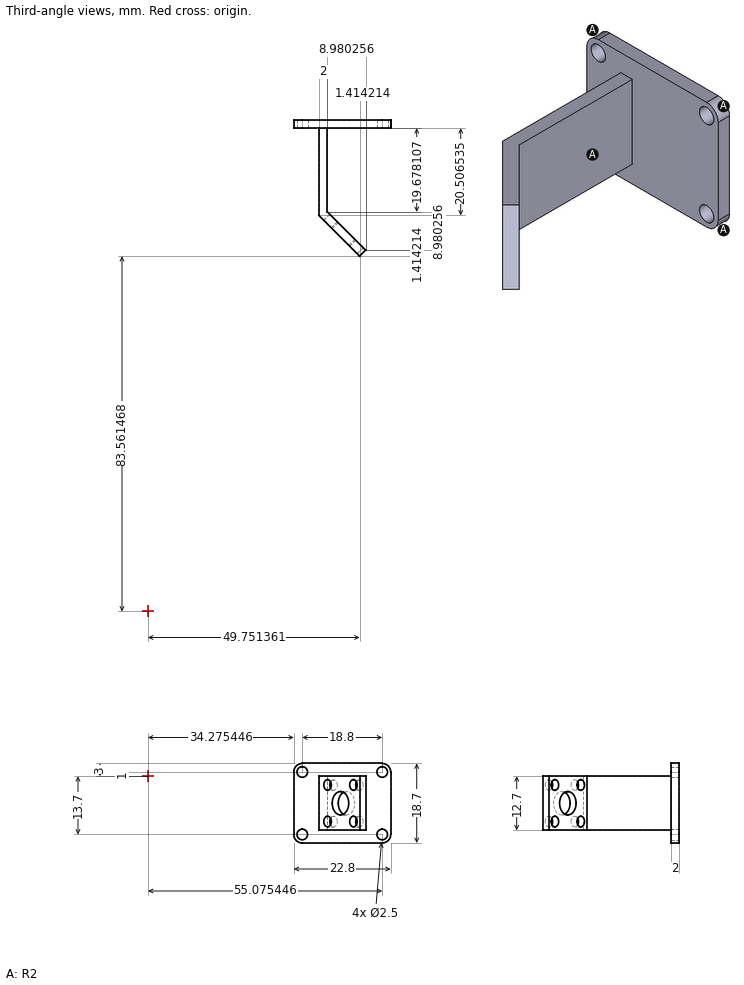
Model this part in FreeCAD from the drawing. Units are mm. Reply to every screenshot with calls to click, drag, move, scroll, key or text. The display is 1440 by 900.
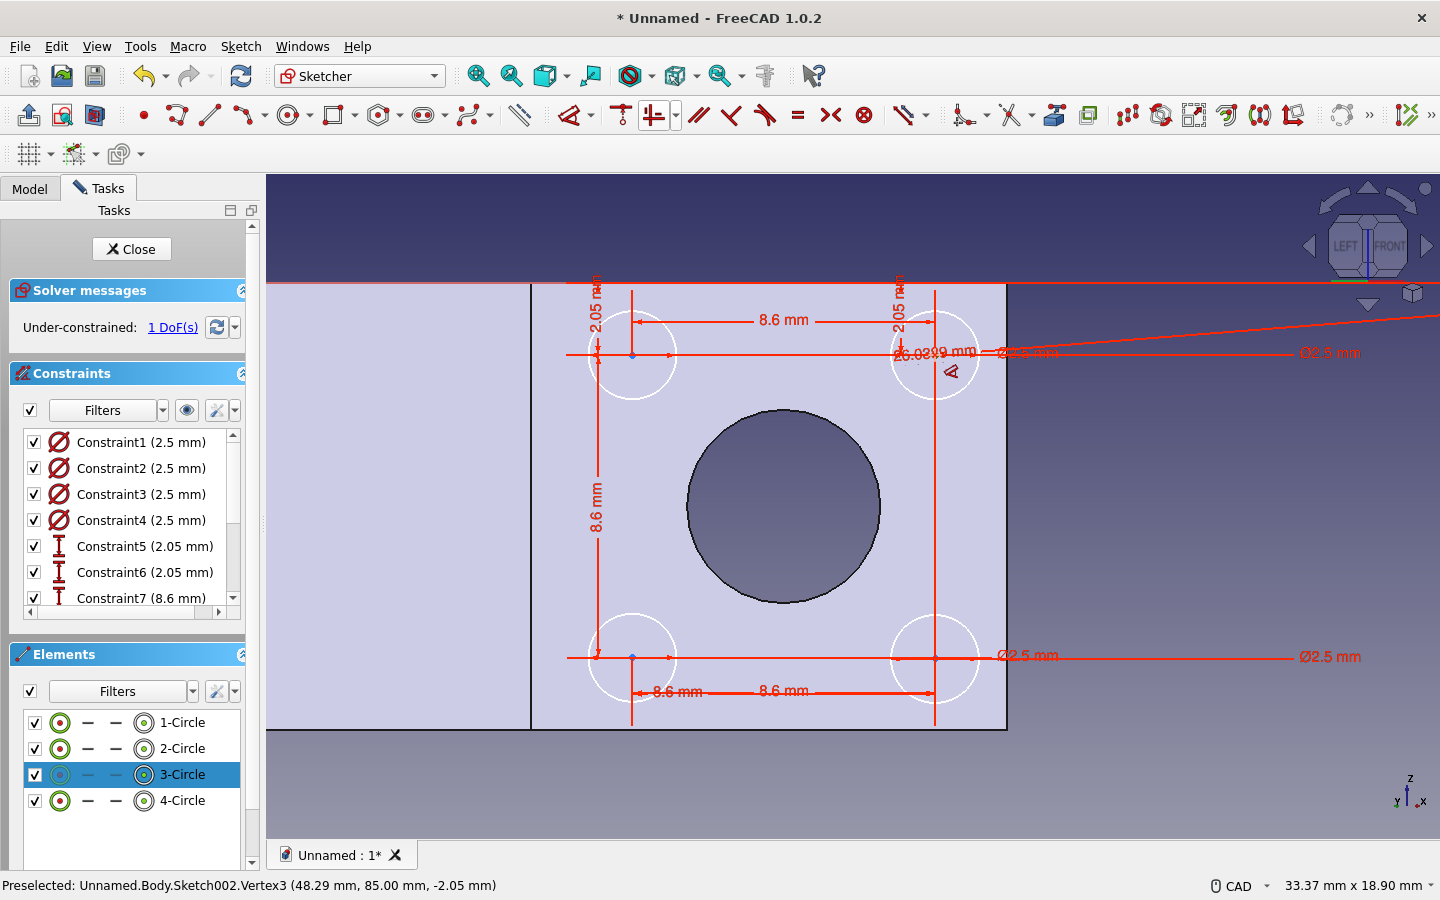
click(935, 659)
click(969, 507)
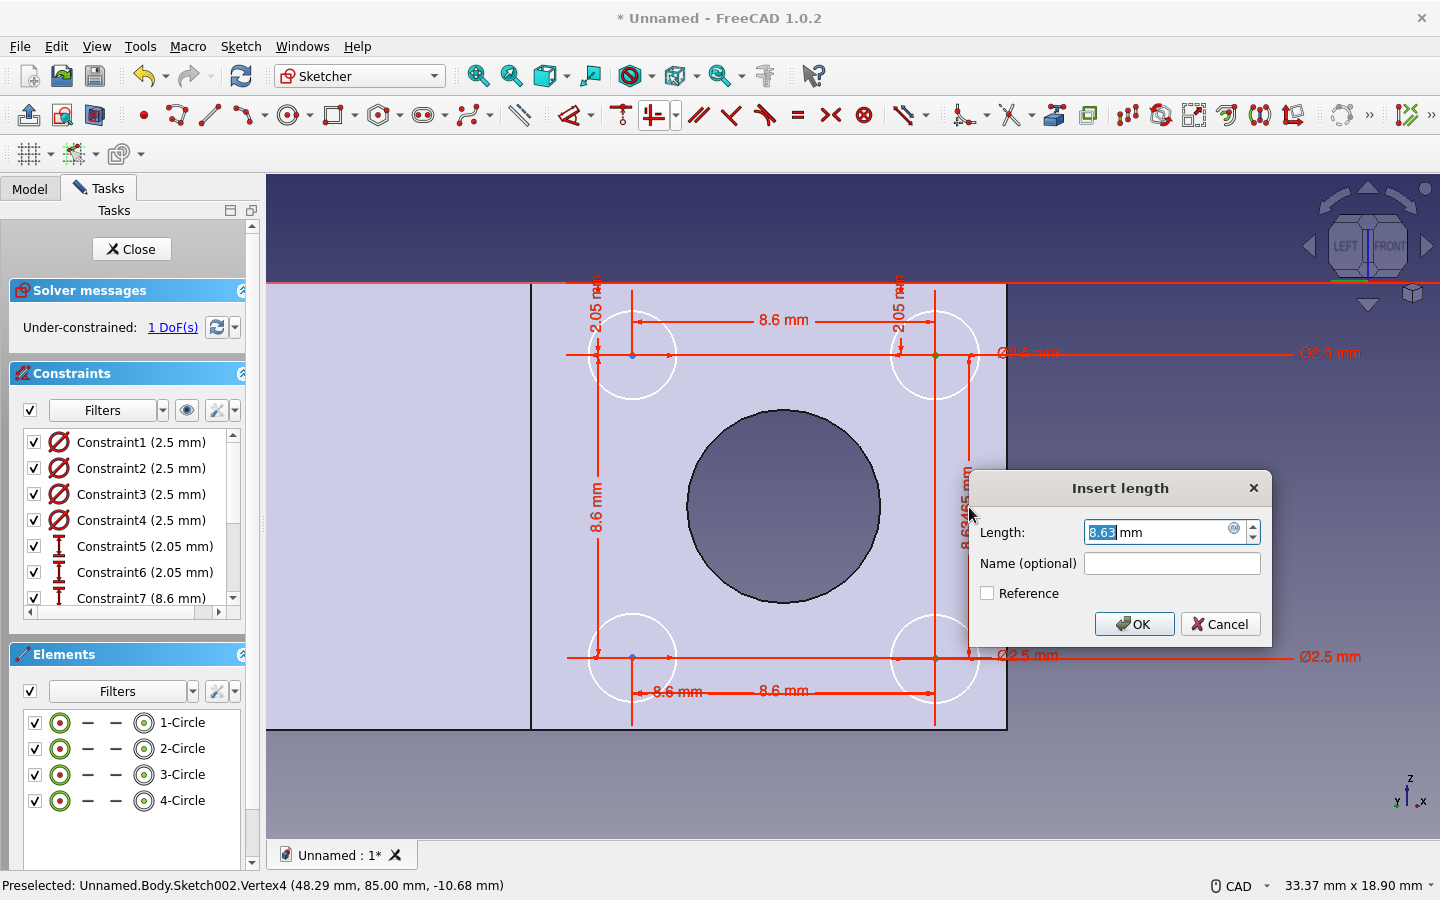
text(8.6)
key(Return)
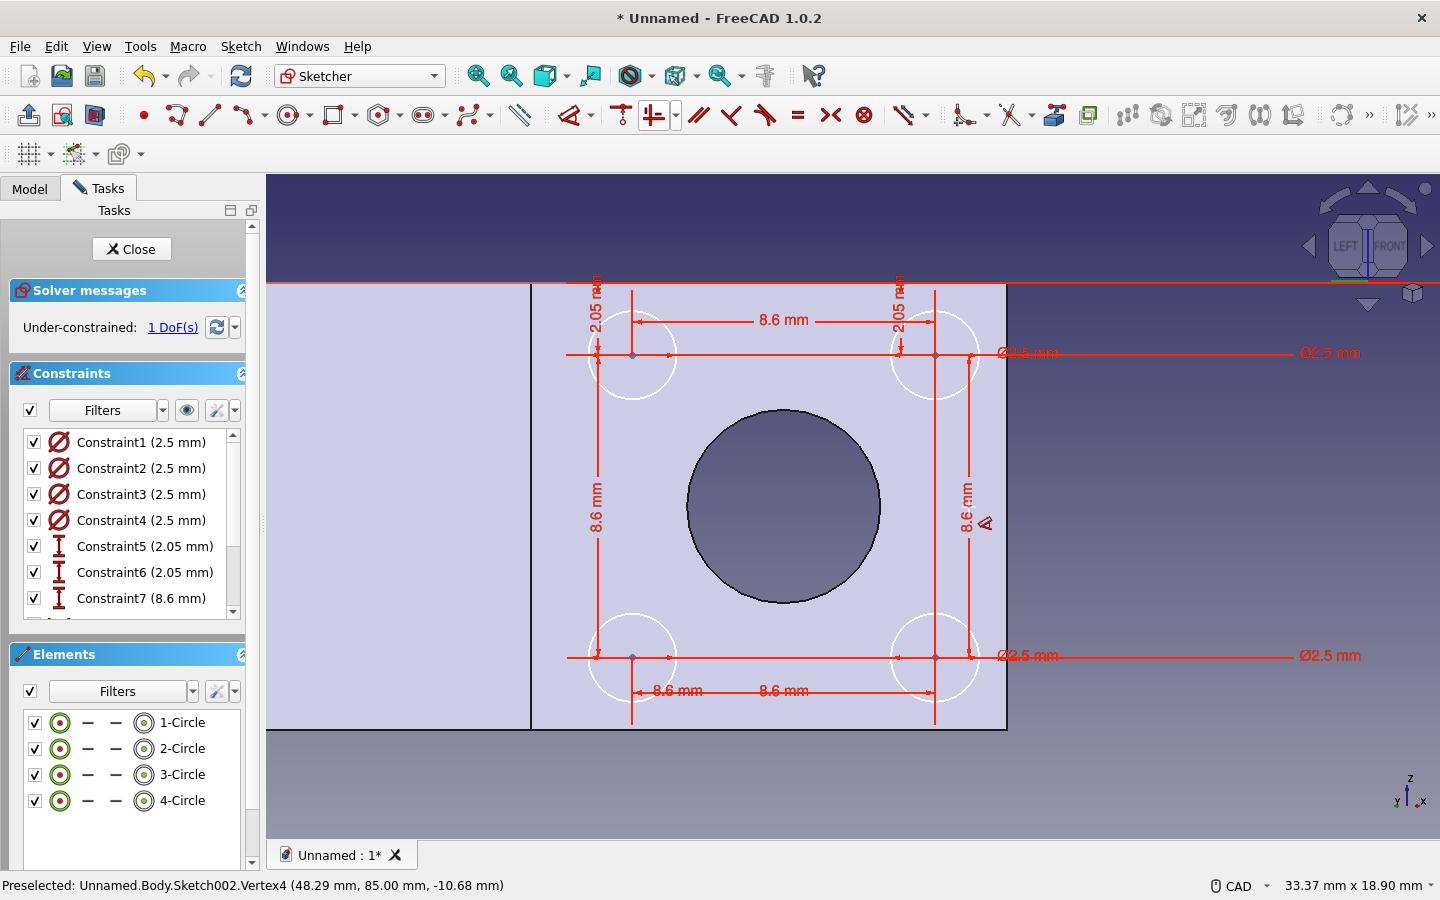
click(632, 658)
click(954, 249)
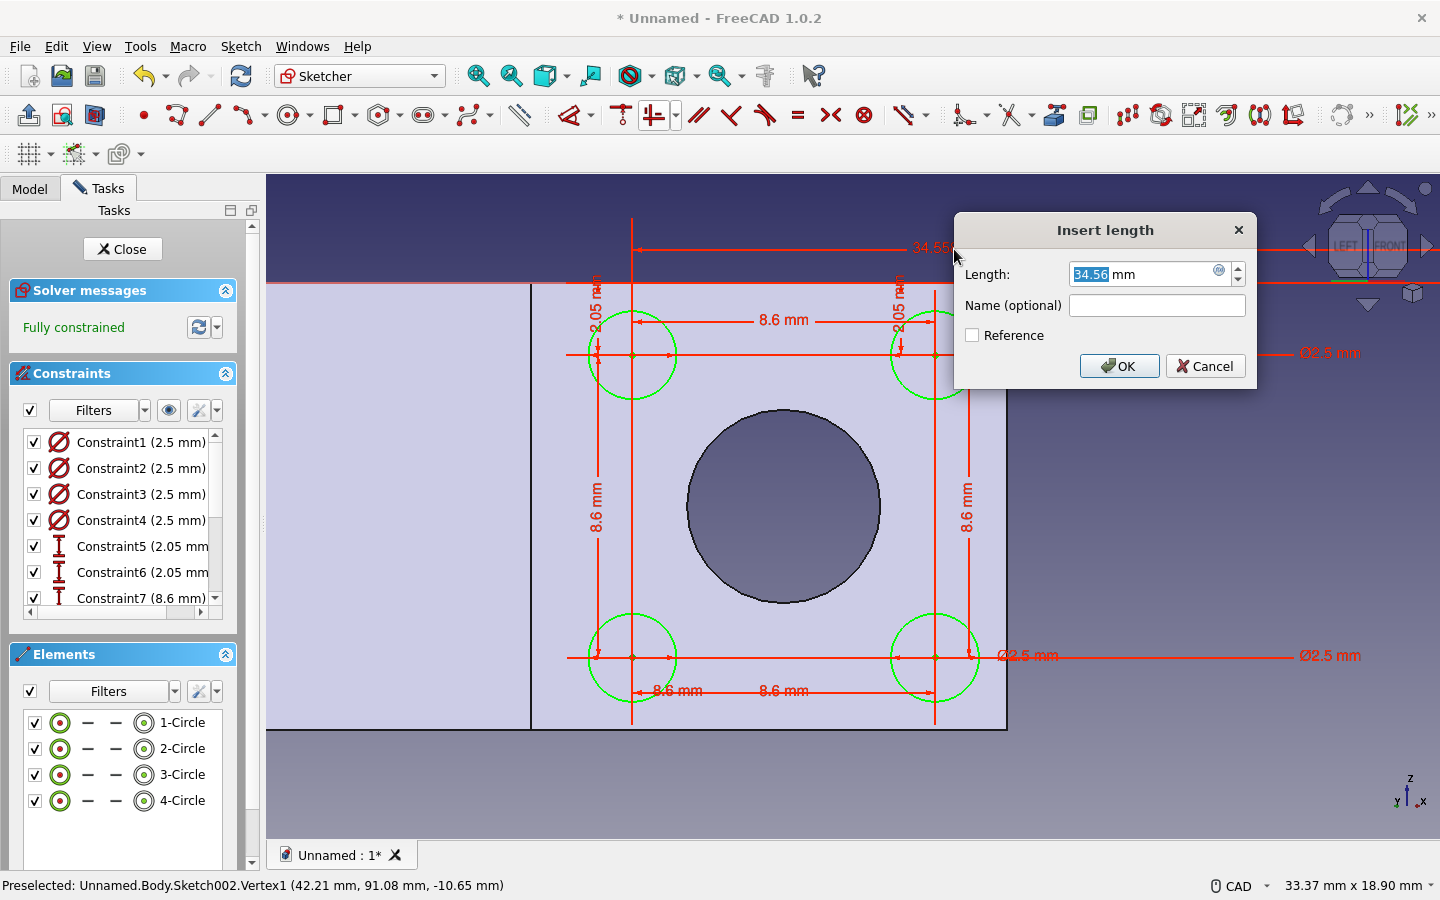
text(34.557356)
key(Return)
key(Escape)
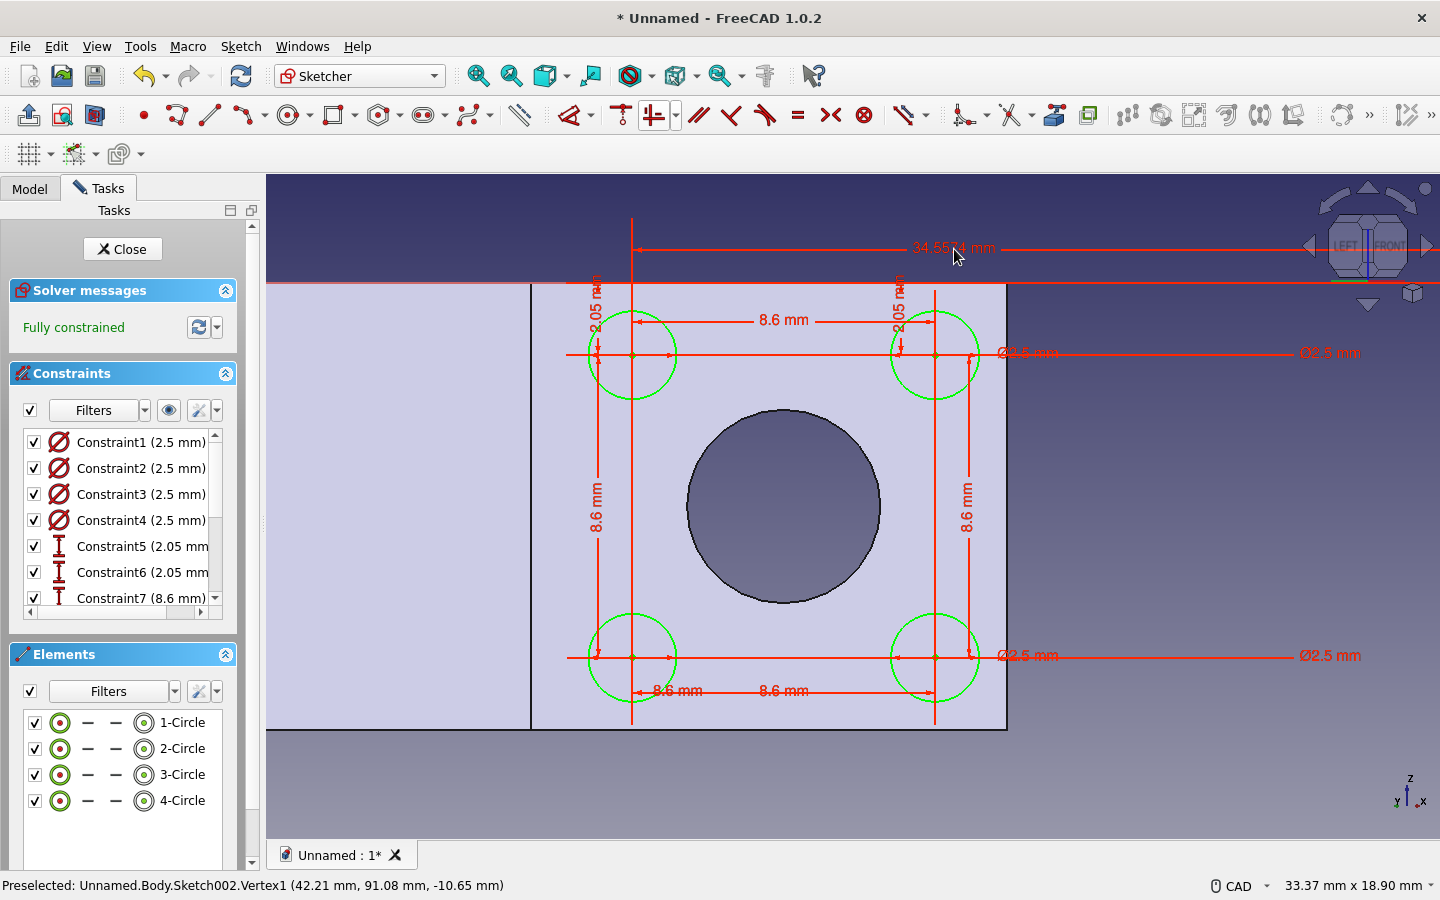
click(123, 249)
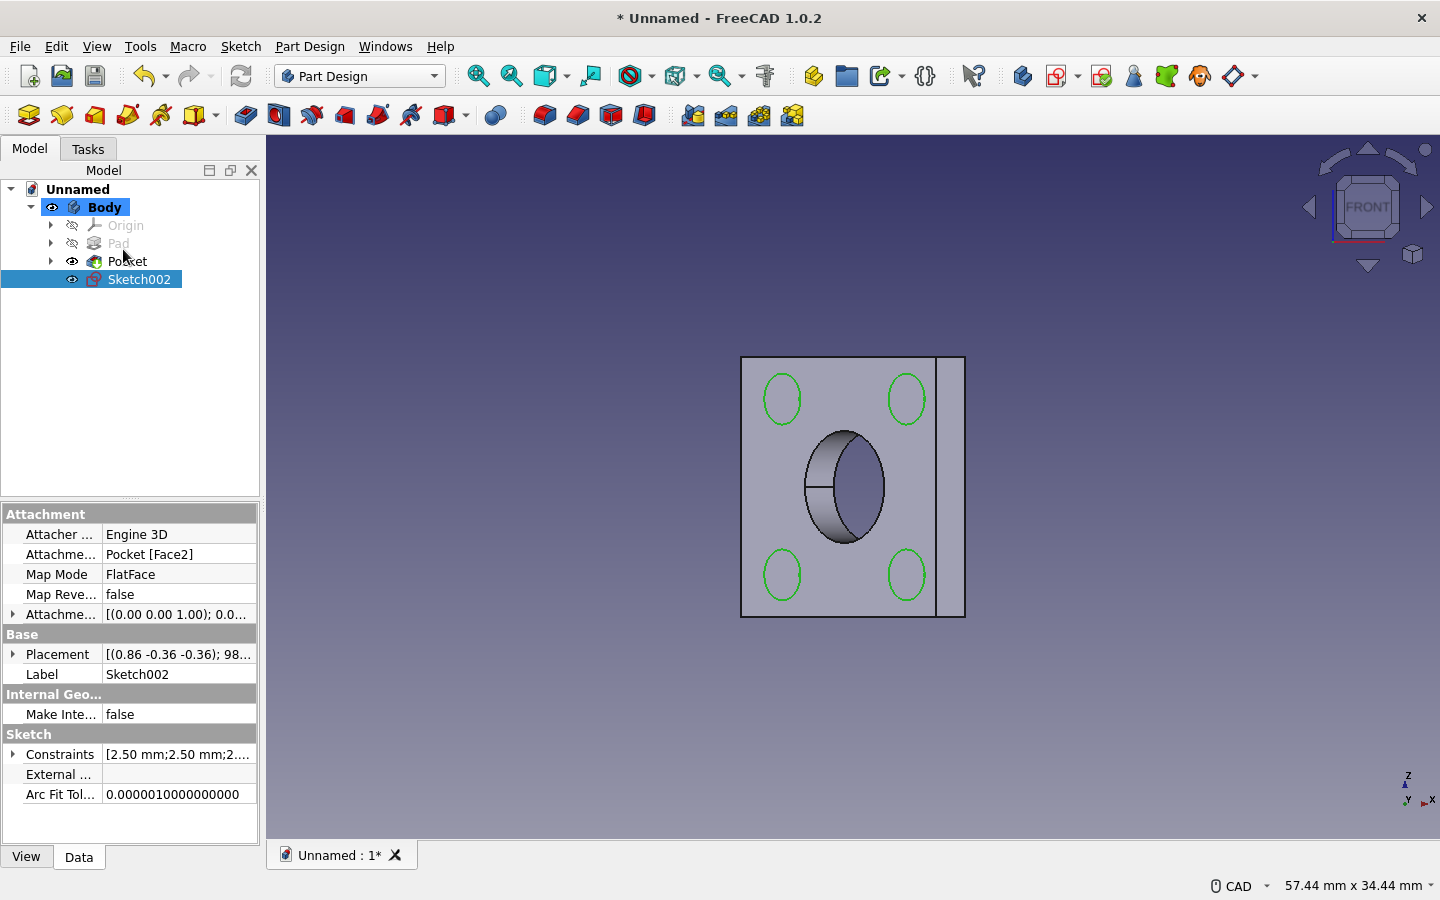
click(246, 116)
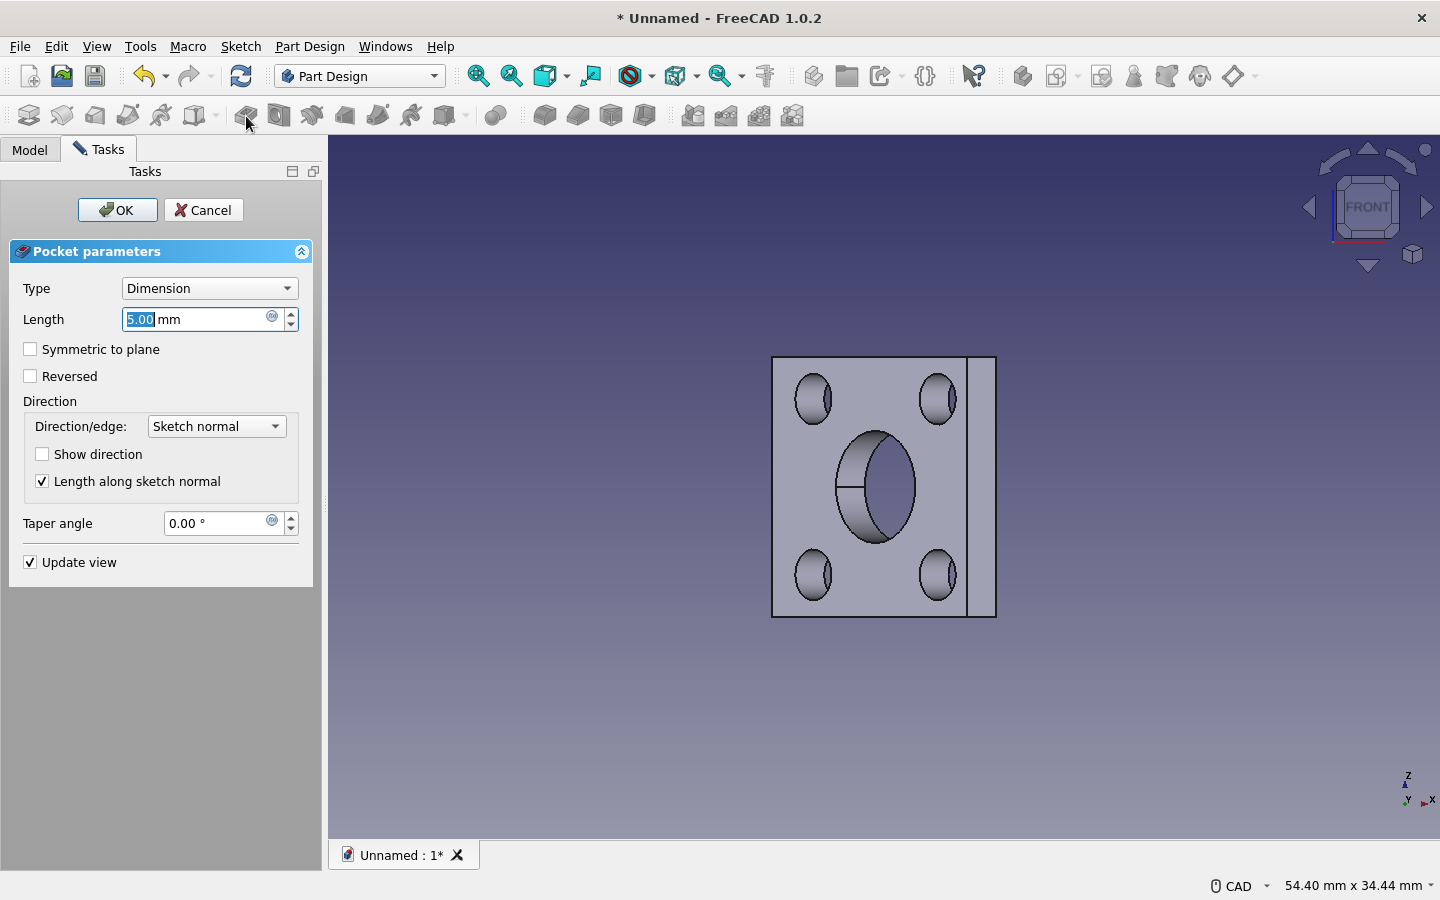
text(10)
key(Tab)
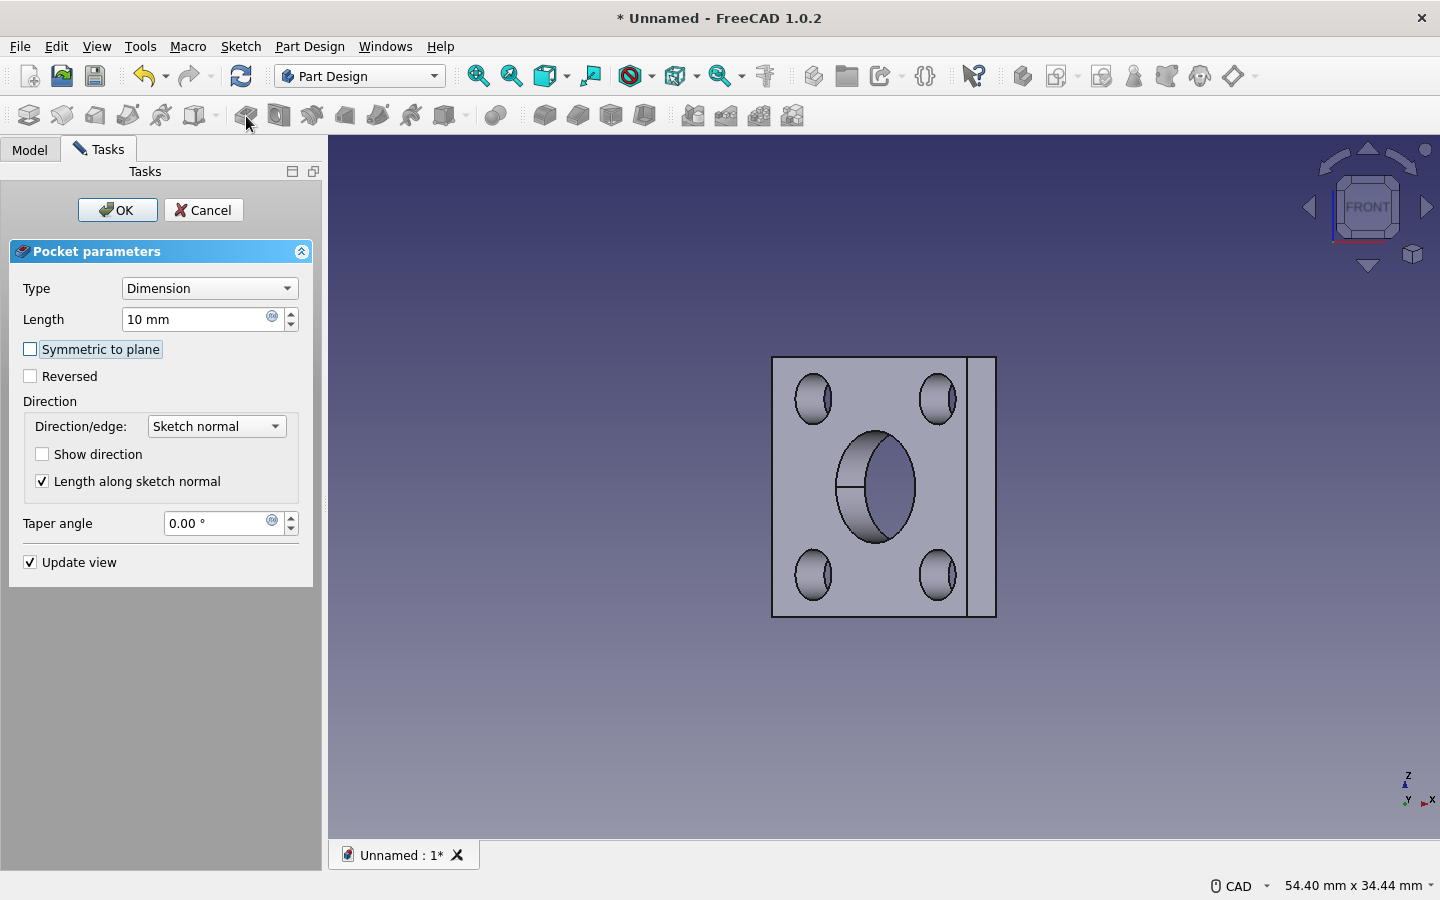
click(118, 210)